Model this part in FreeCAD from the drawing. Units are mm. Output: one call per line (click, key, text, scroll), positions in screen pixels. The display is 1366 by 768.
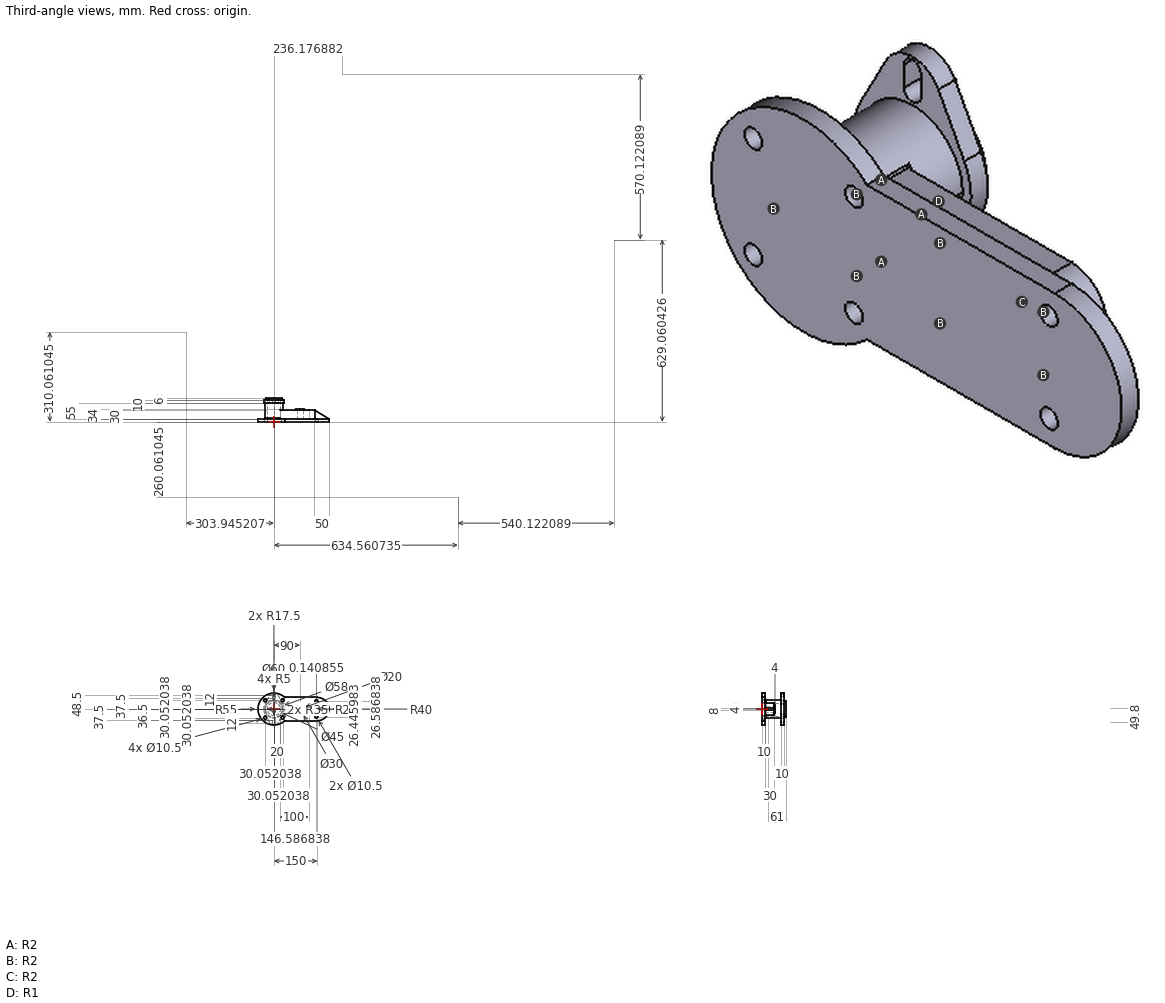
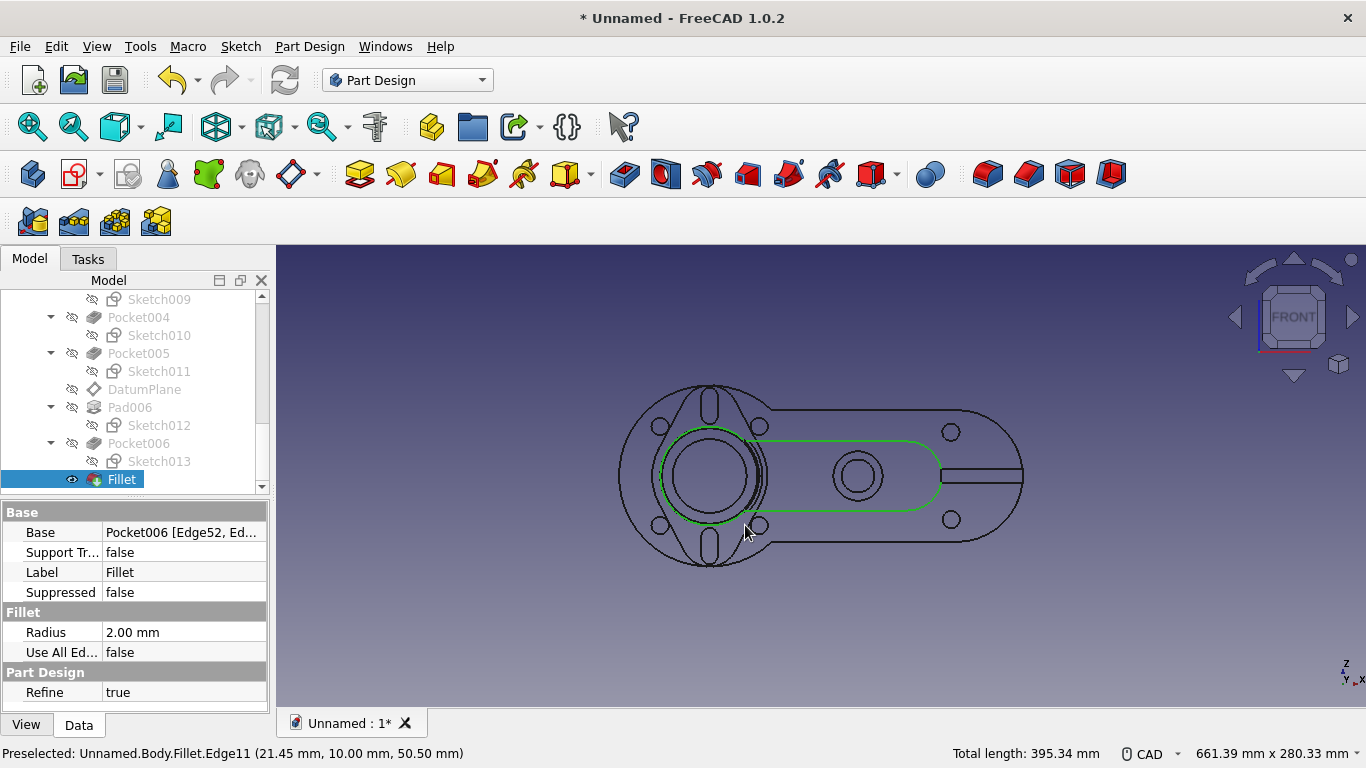
key(v)
key(f)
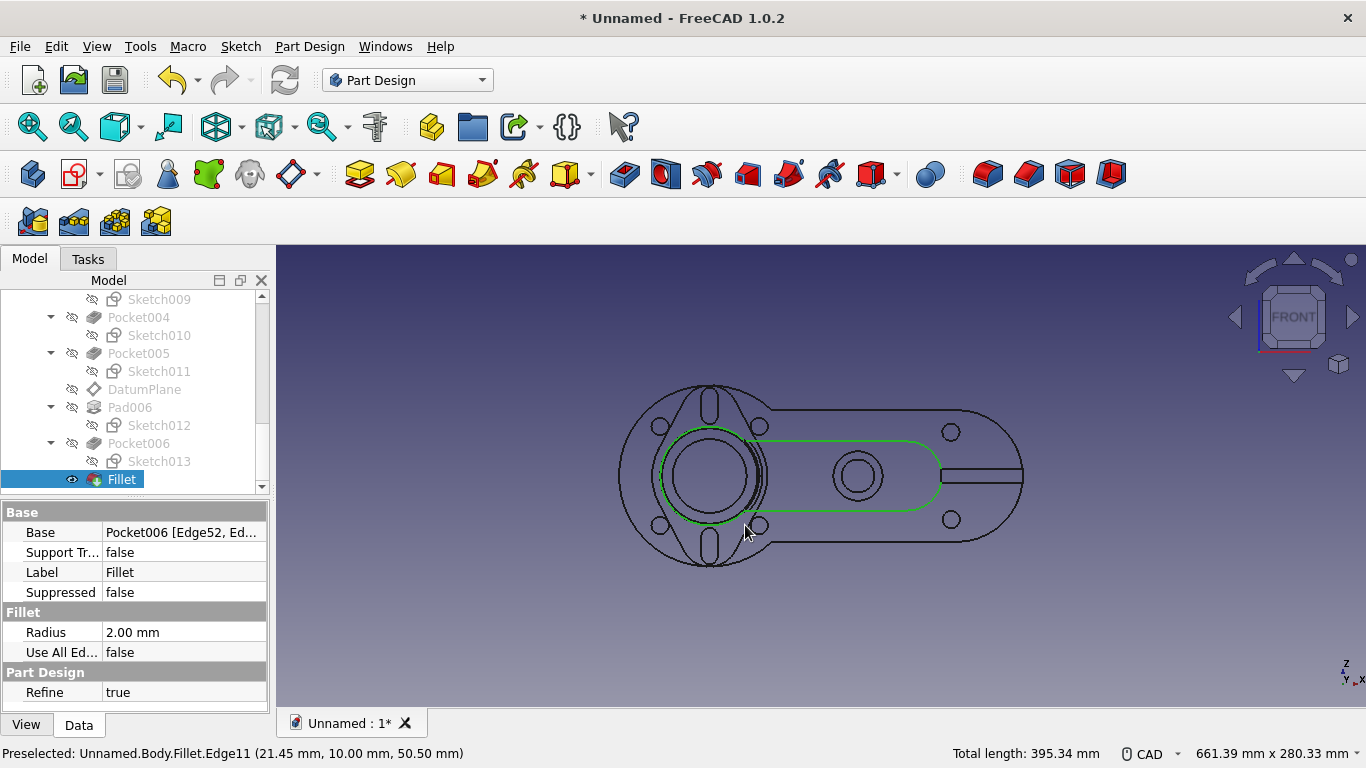
scroll(745, 440, up, 14)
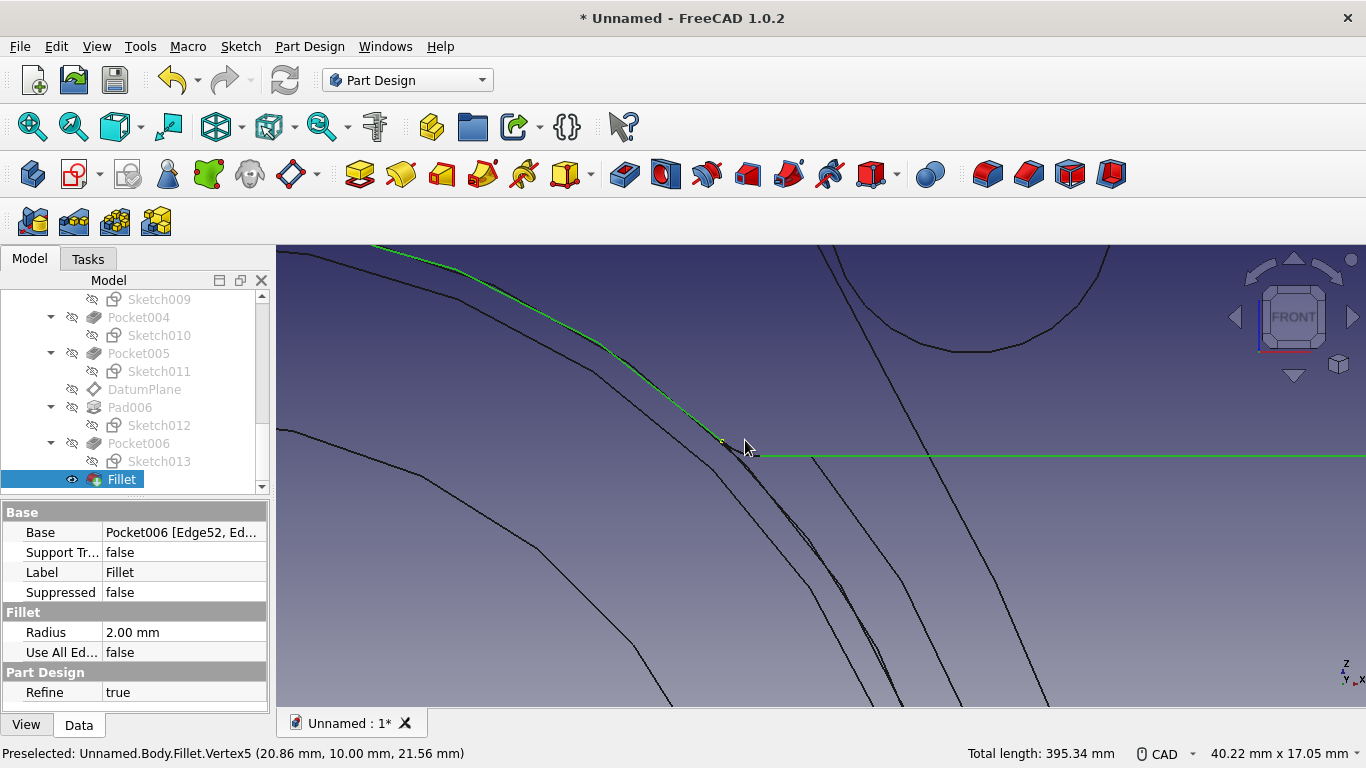
click(740, 451, ctrl)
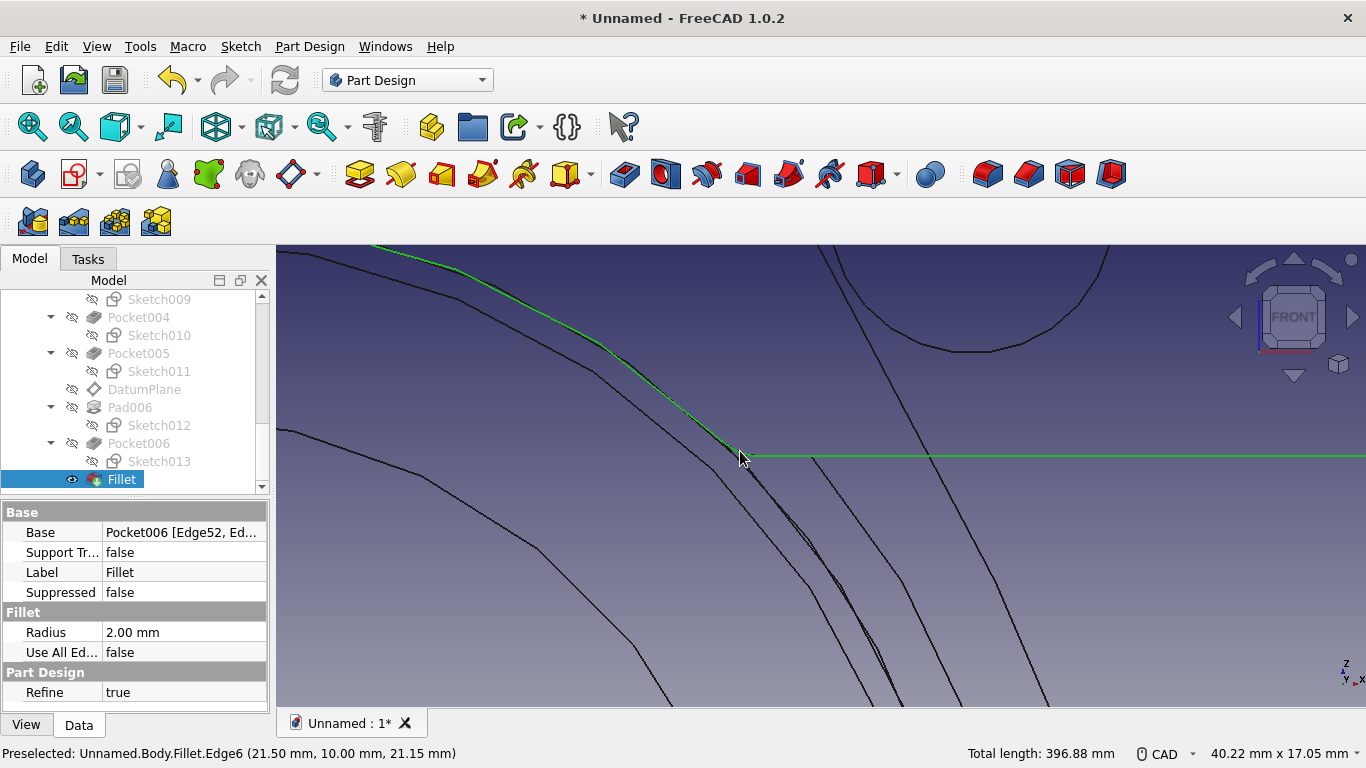
key(v)
key(1)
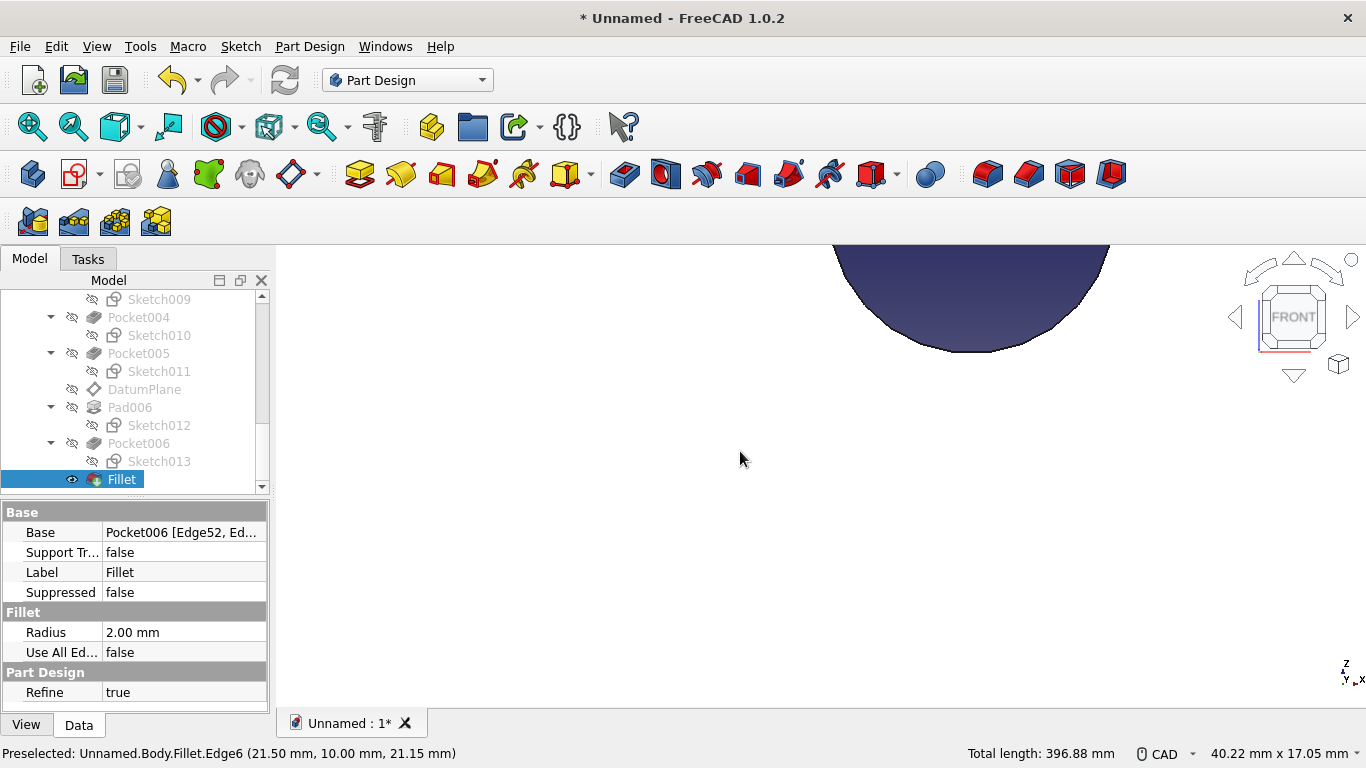
click(988, 174)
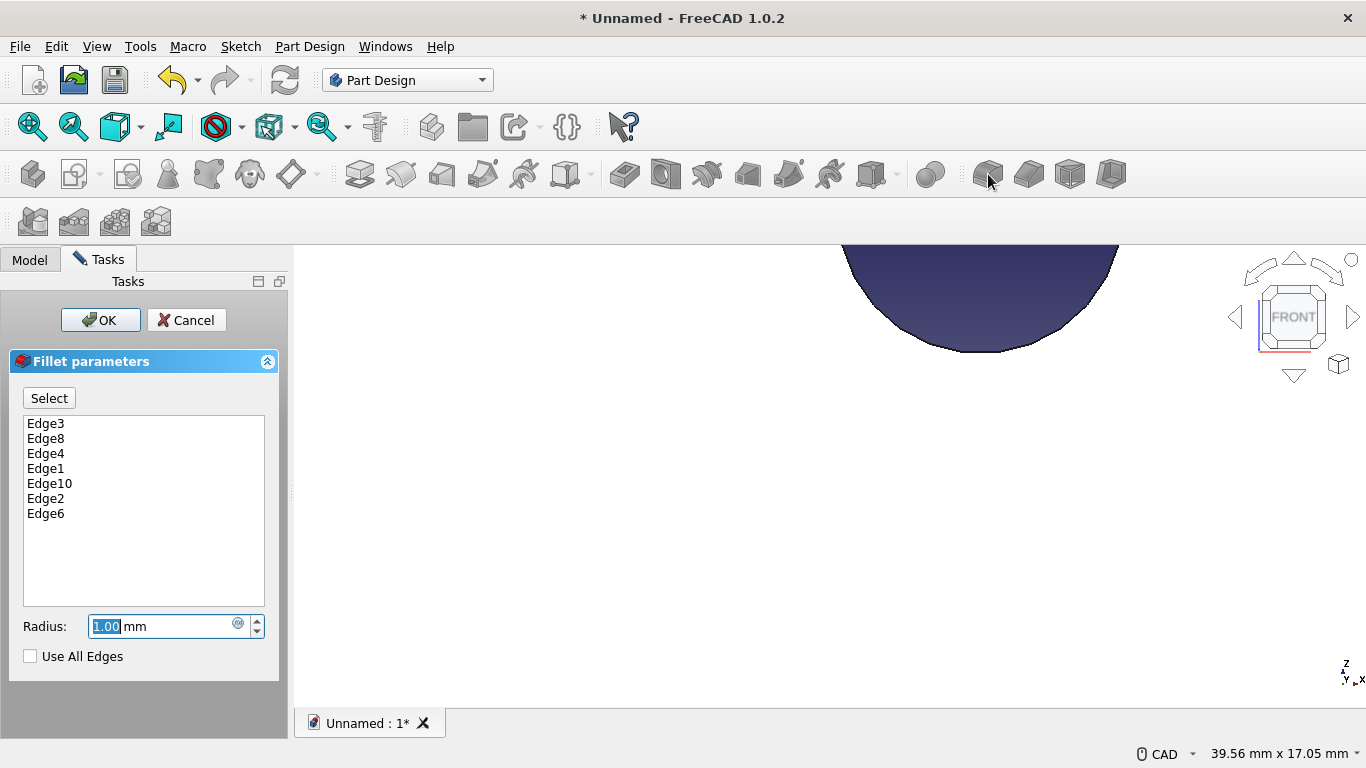
text(2)
key(Tab)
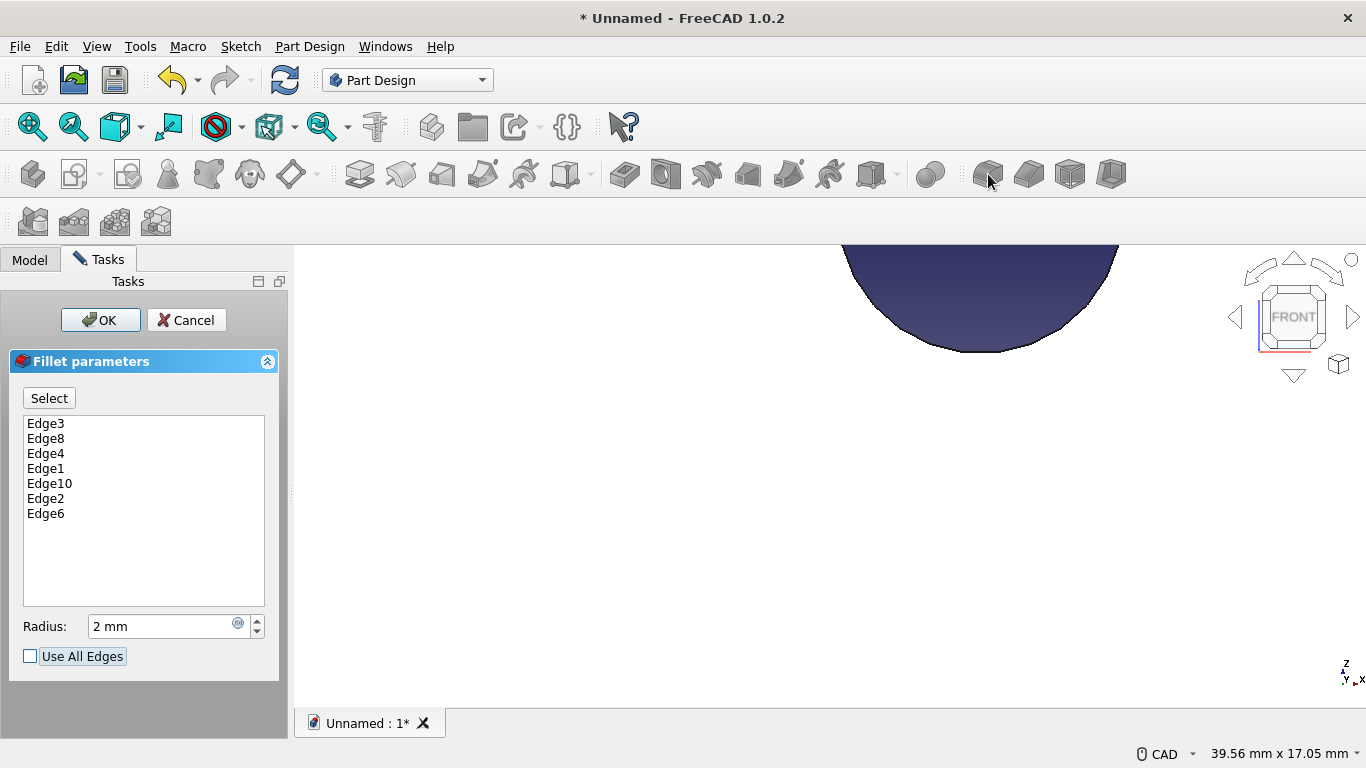
click(101, 320)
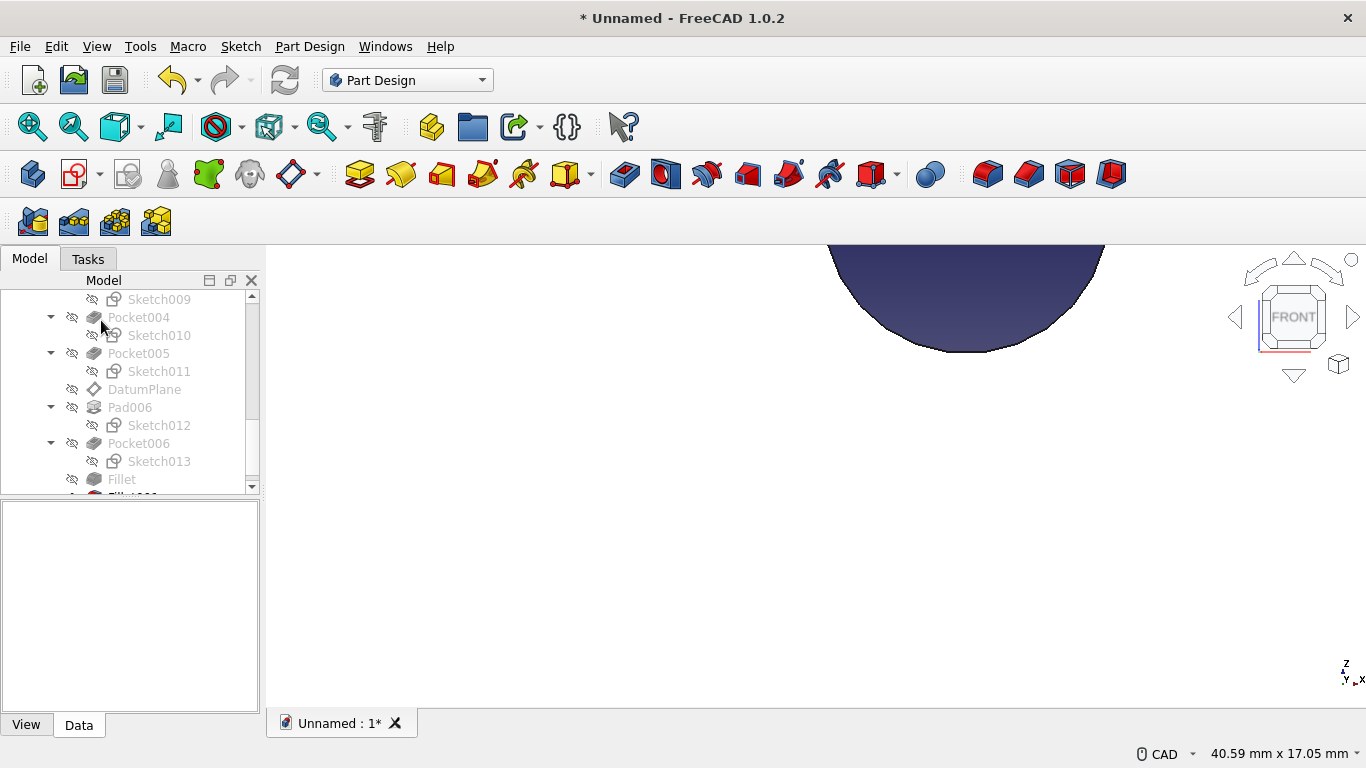
key(v)
key(f)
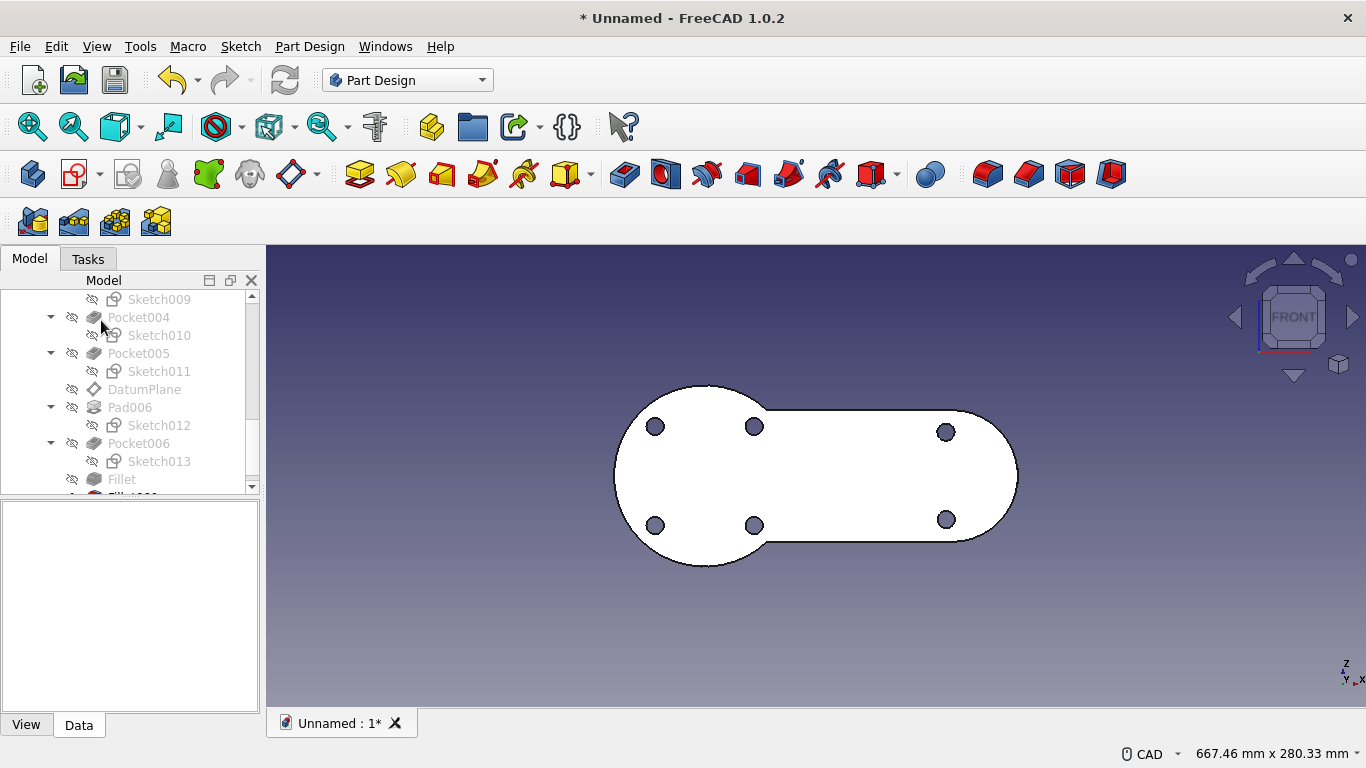
key(0)